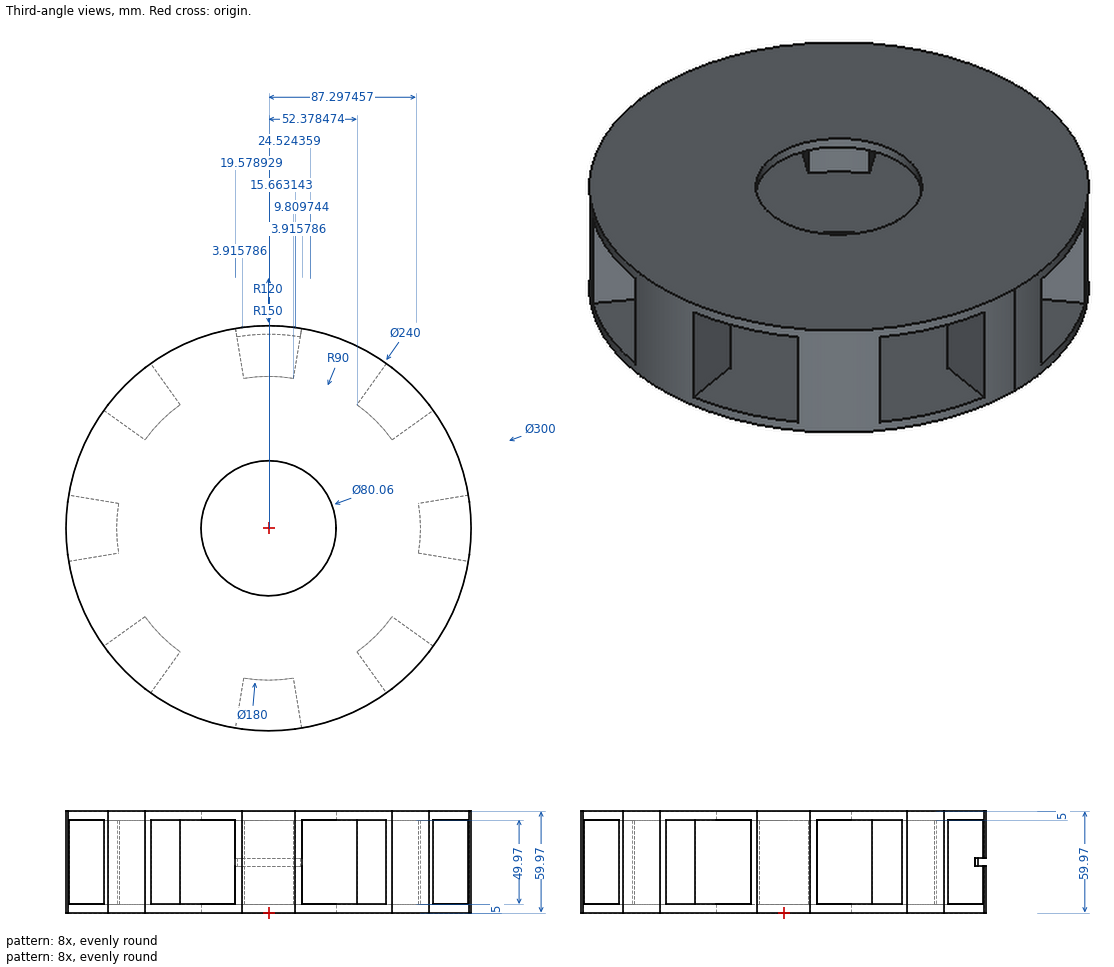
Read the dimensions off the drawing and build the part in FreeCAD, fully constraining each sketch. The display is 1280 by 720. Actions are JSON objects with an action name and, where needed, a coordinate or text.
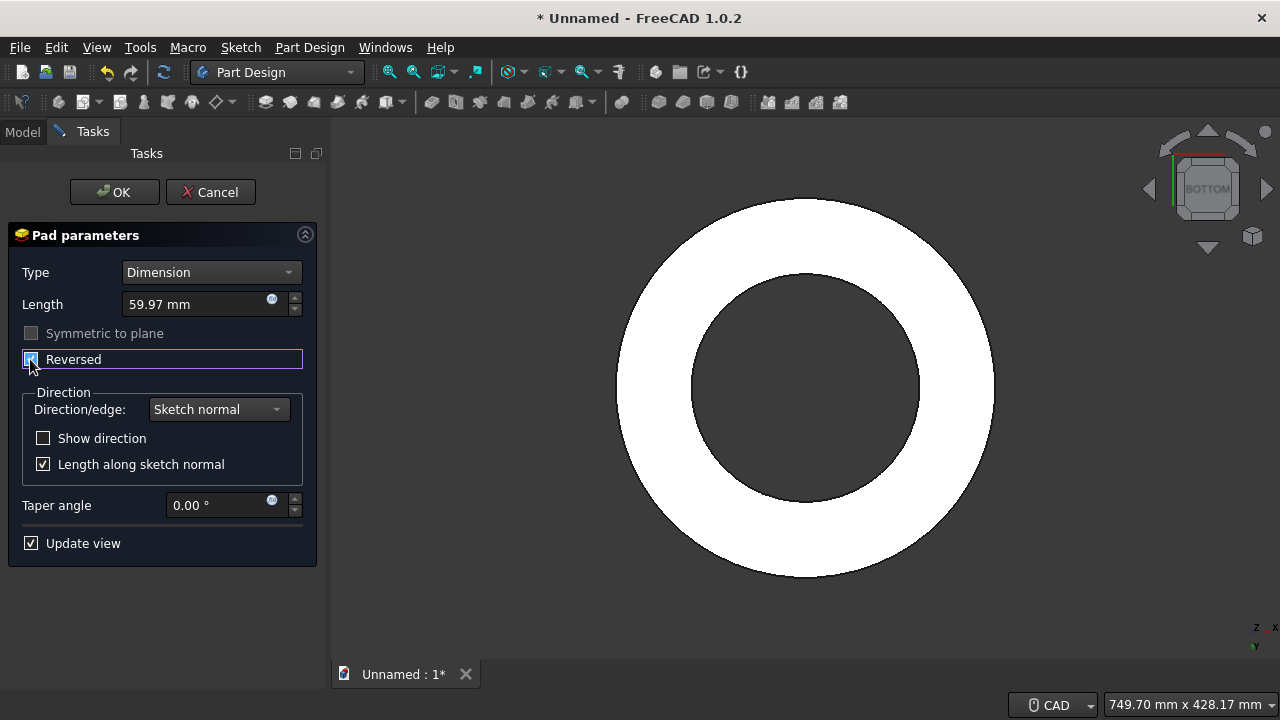
{"action": "left_click", "coordinate": [115, 192]}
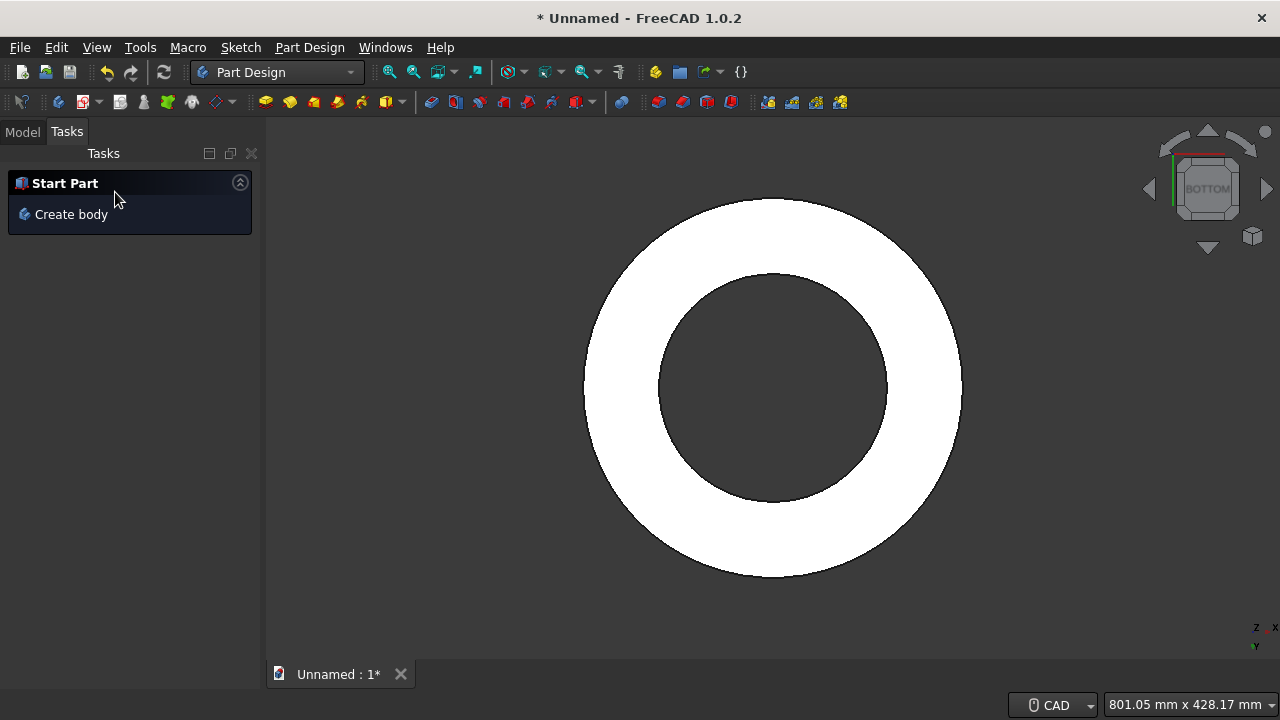
{"action": "left_click", "coordinate": [84, 102]}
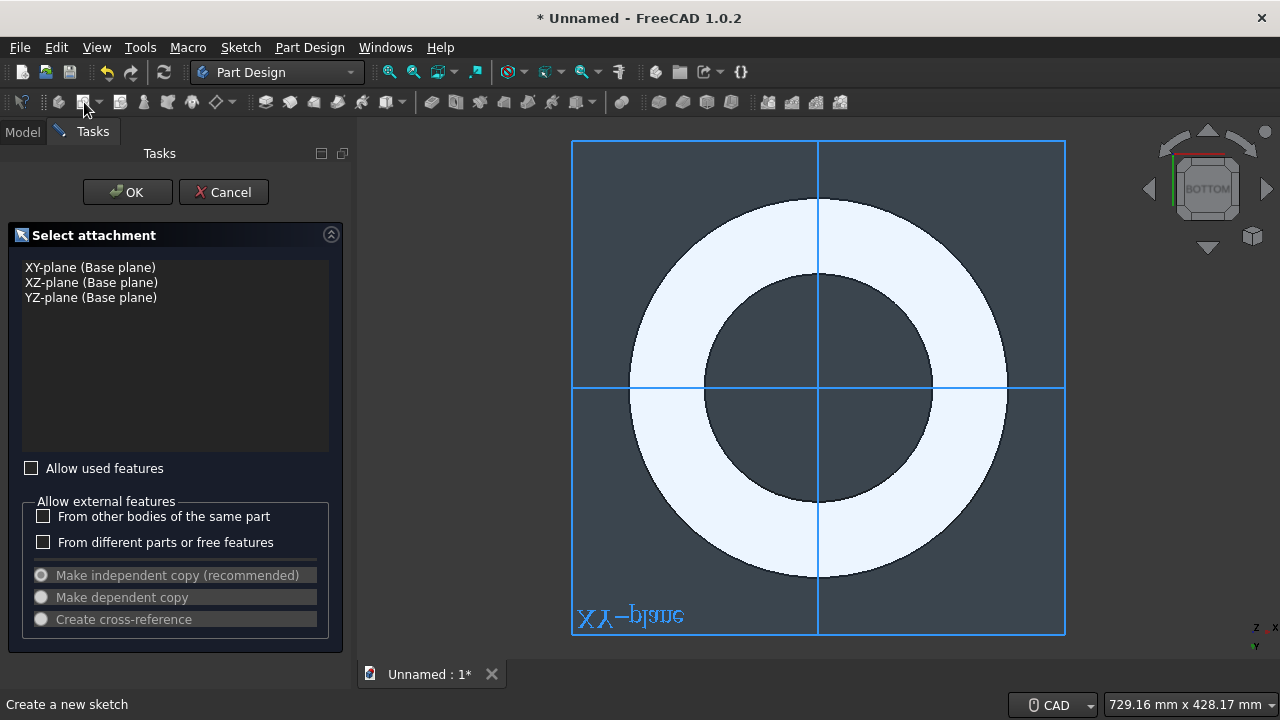
{"action": "left_click", "coordinate": [82, 268]}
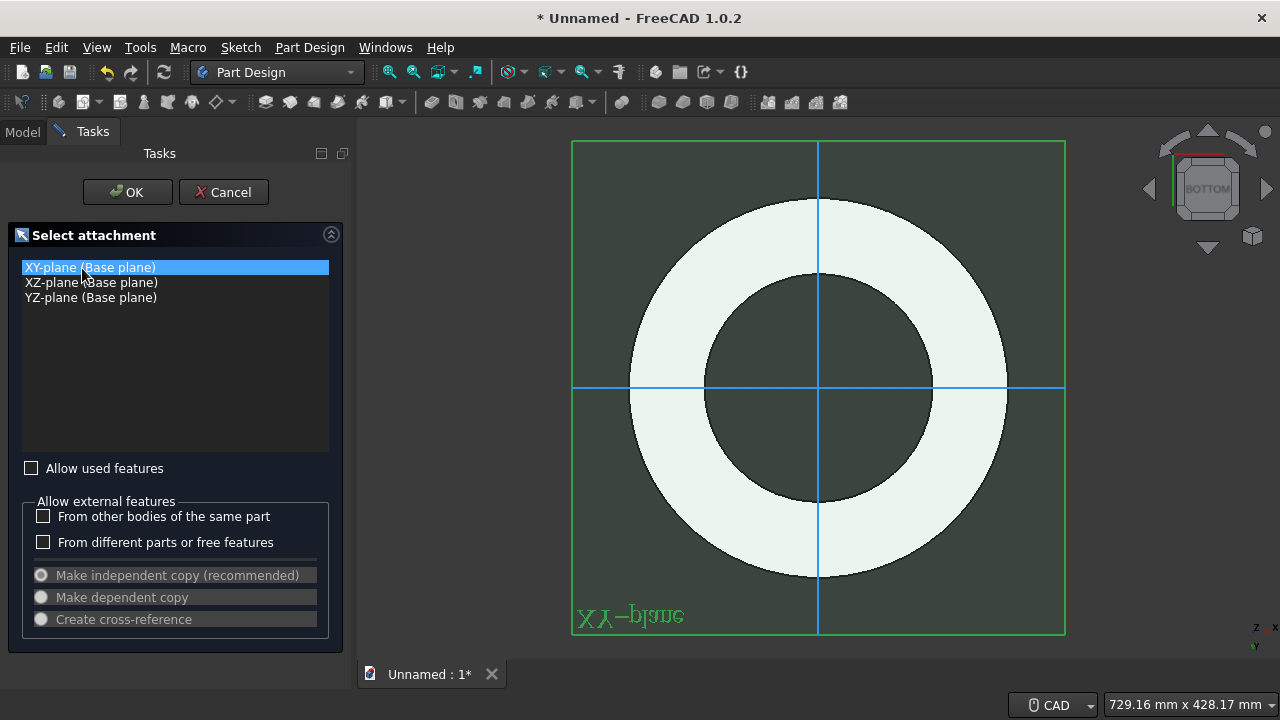
{"action": "left_click", "coordinate": [128, 192]}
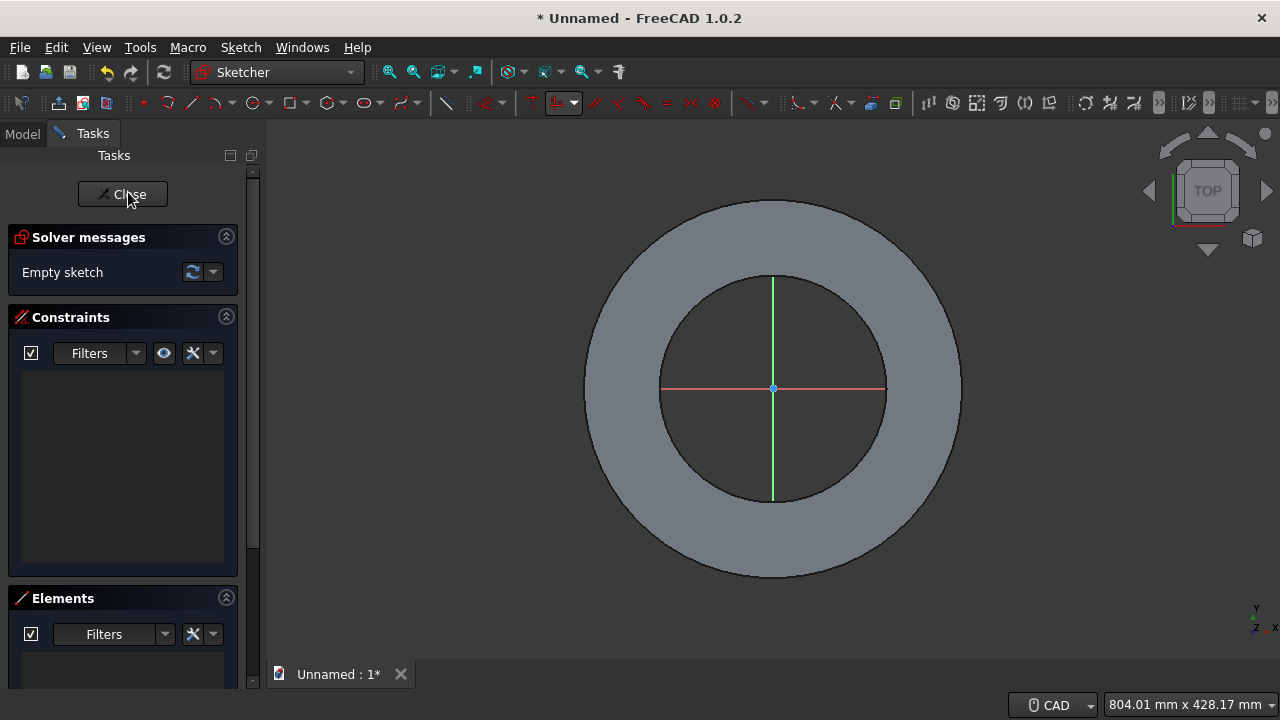
{"action": "left_click", "coordinate": [108, 104]}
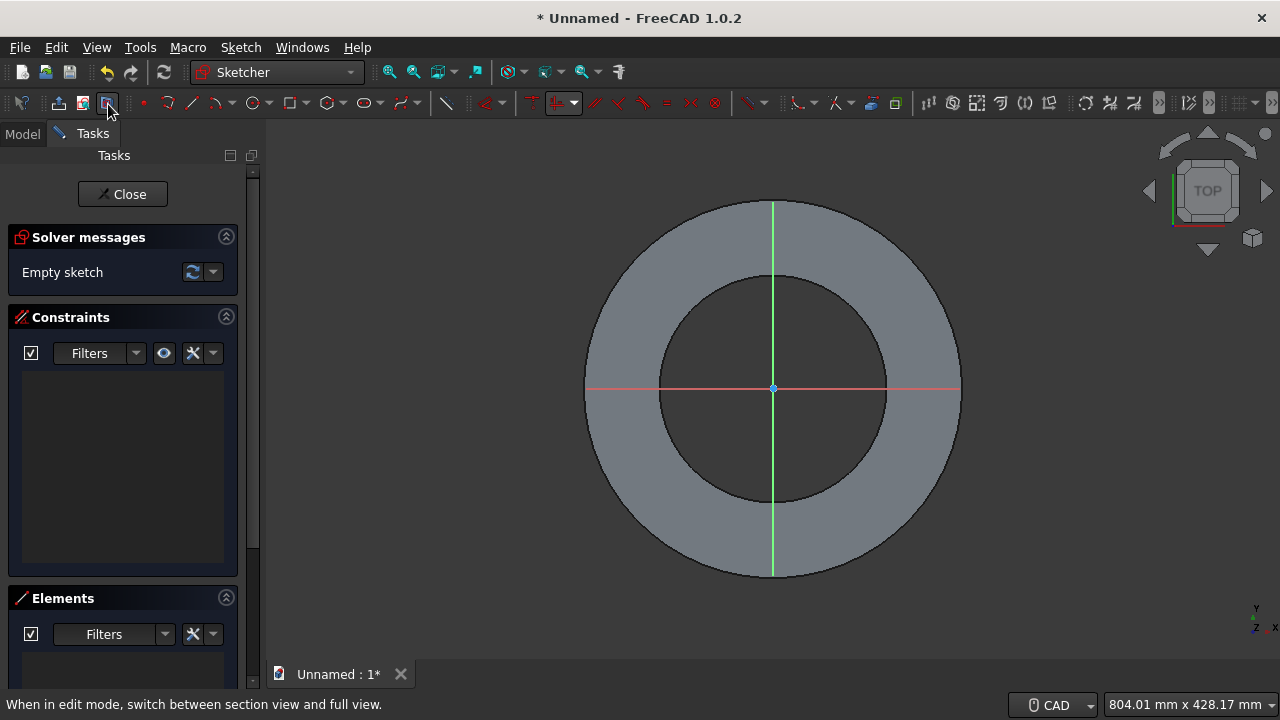
{"action": "scroll", "coordinate": [782, 198], "scroll_direction": "up", "scroll_amount": 11}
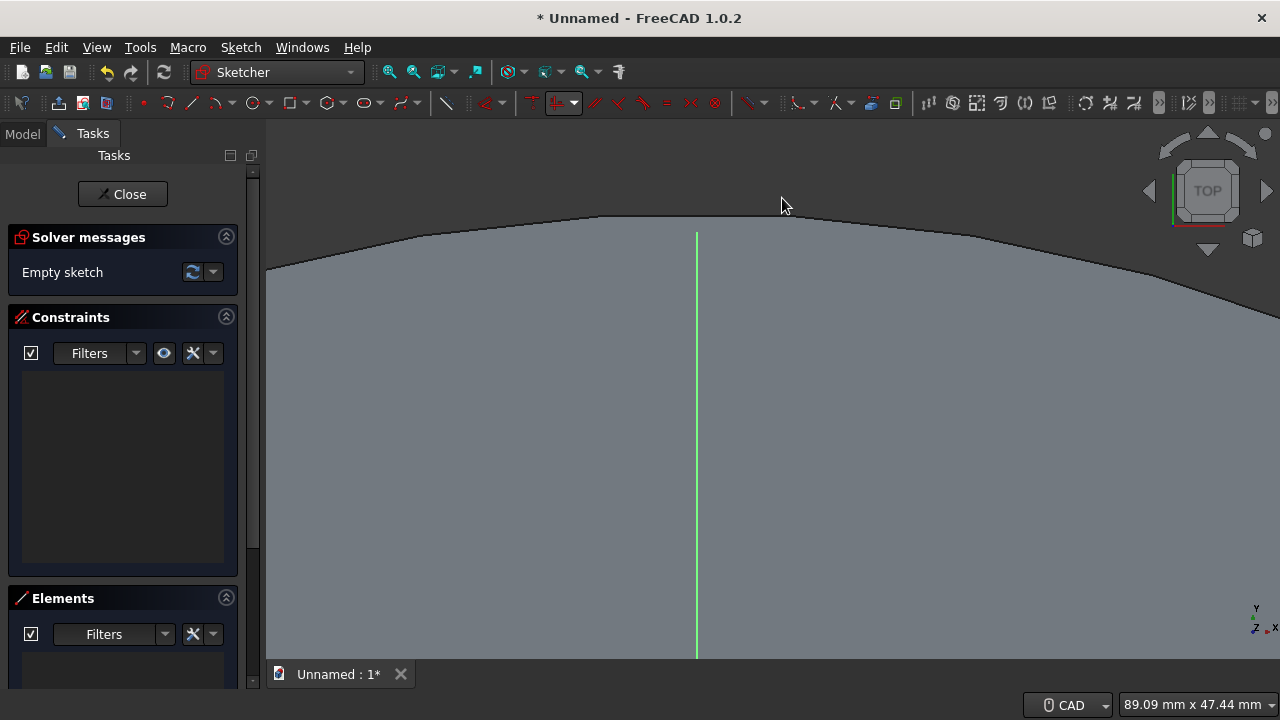
{"action": "left_click", "coordinate": [192, 104]}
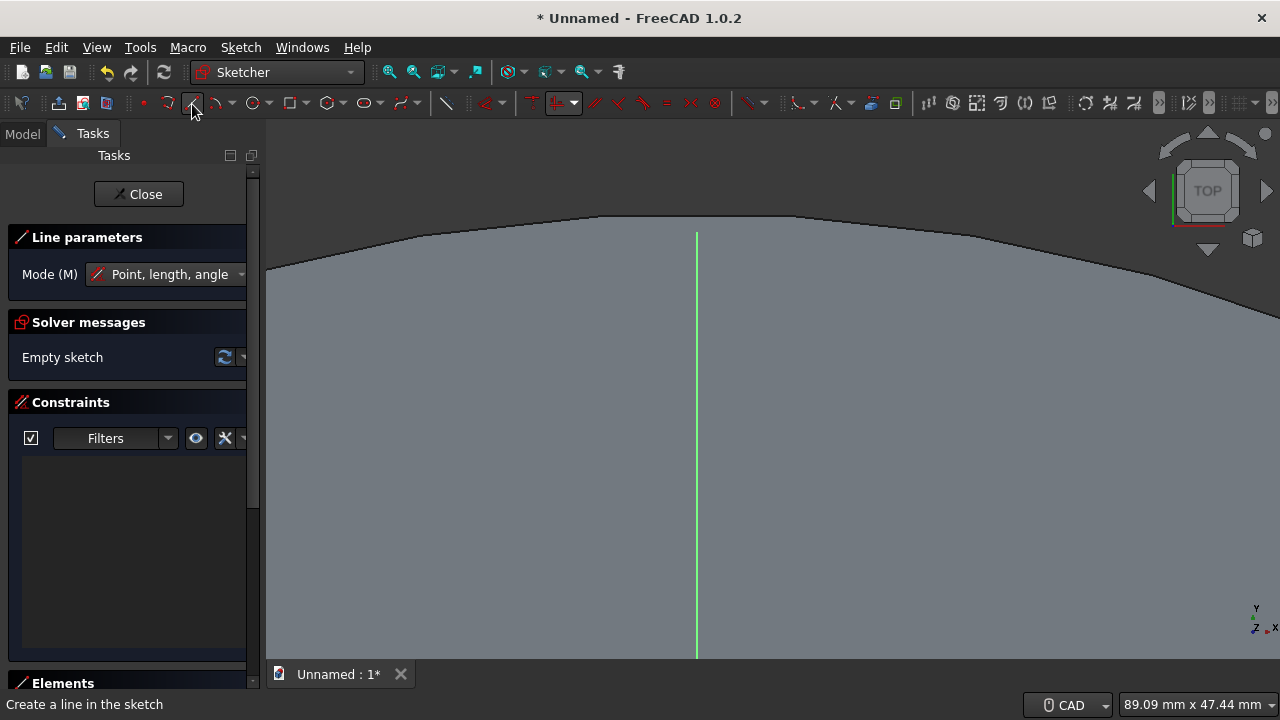
{"action": "left_click", "coordinate": [474, 228]}
{"action": "left_click", "coordinate": [518, 566]}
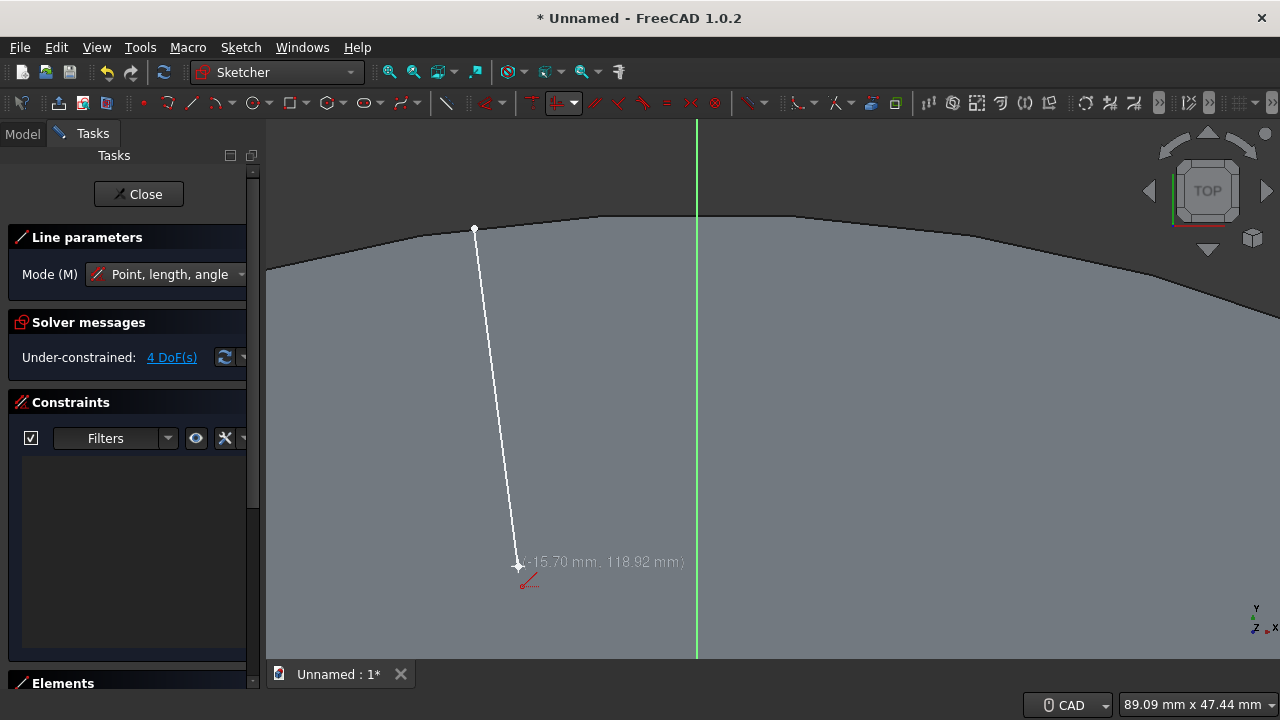
{"action": "left_click", "coordinate": [875, 566]}
{"action": "left_click", "coordinate": [920, 228]}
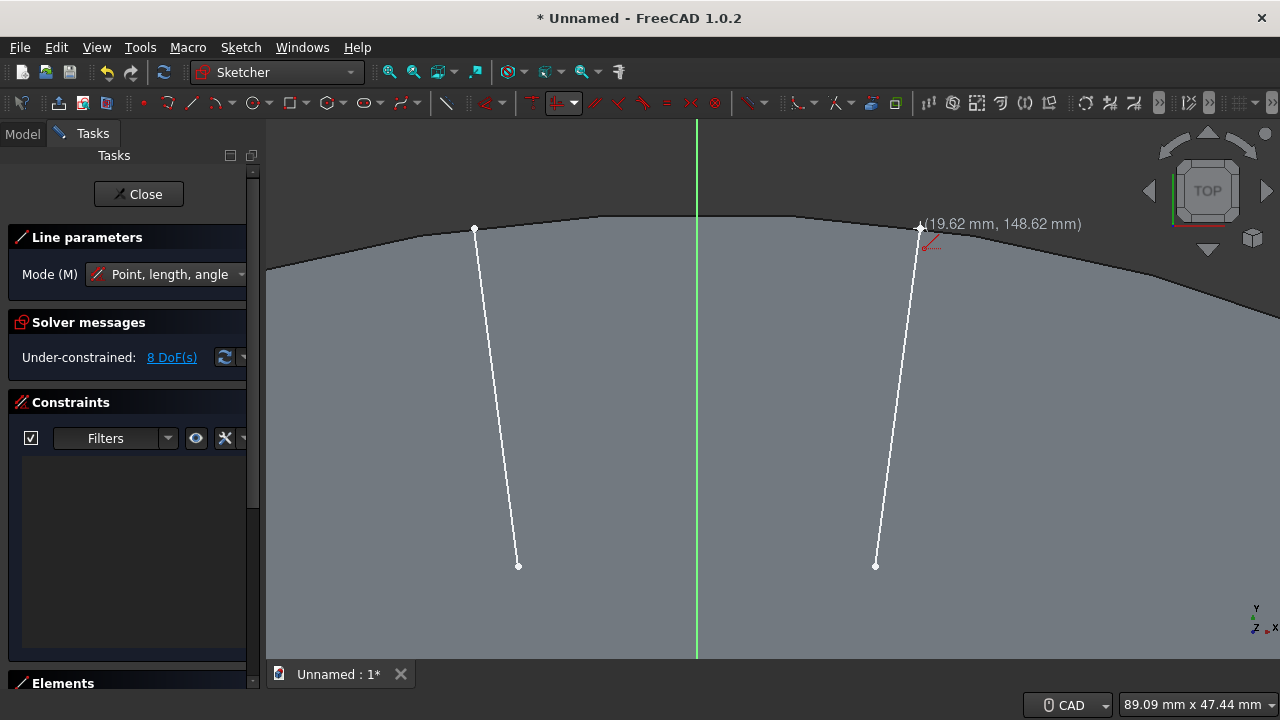
{"action": "key", "text": "g 3 a"}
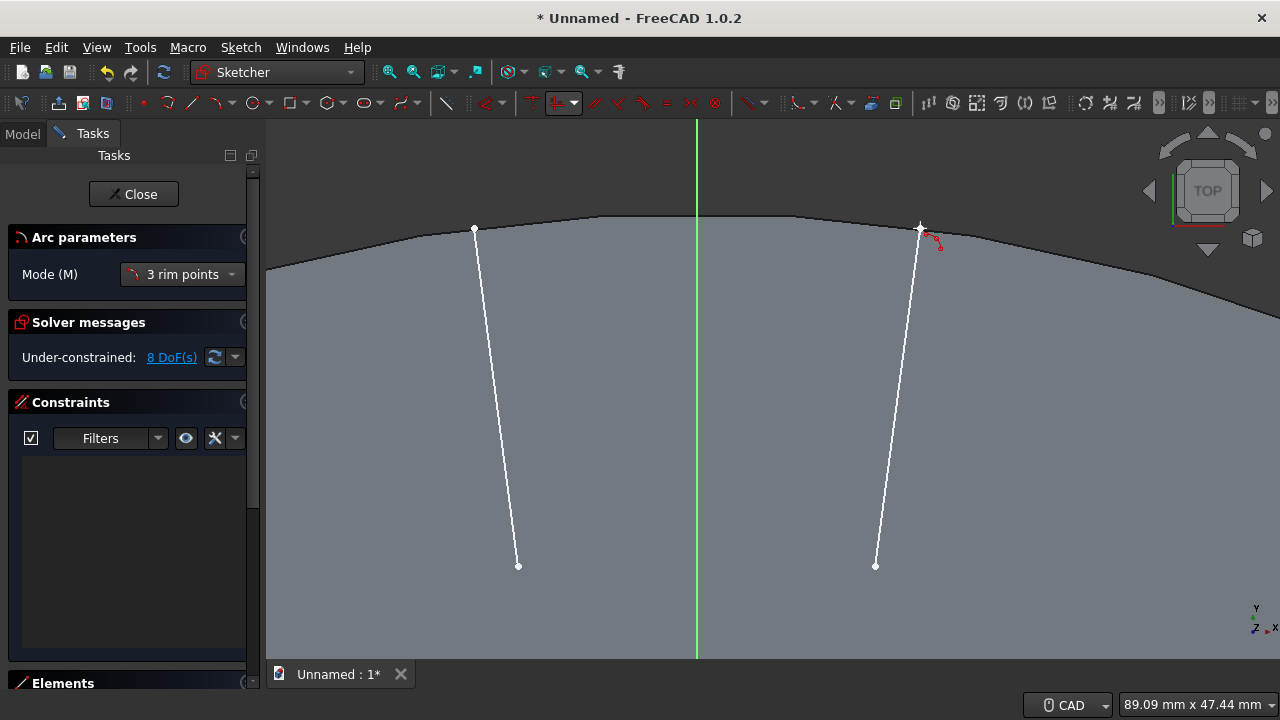
{"action": "left_click", "coordinate": [518, 567]}
{"action": "left_click", "coordinate": [875, 567]}